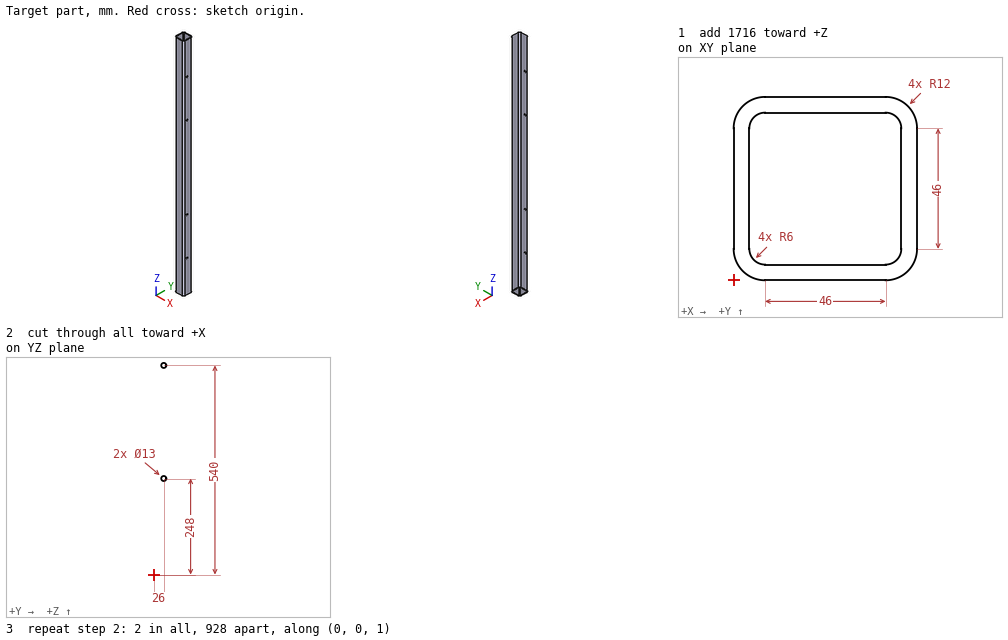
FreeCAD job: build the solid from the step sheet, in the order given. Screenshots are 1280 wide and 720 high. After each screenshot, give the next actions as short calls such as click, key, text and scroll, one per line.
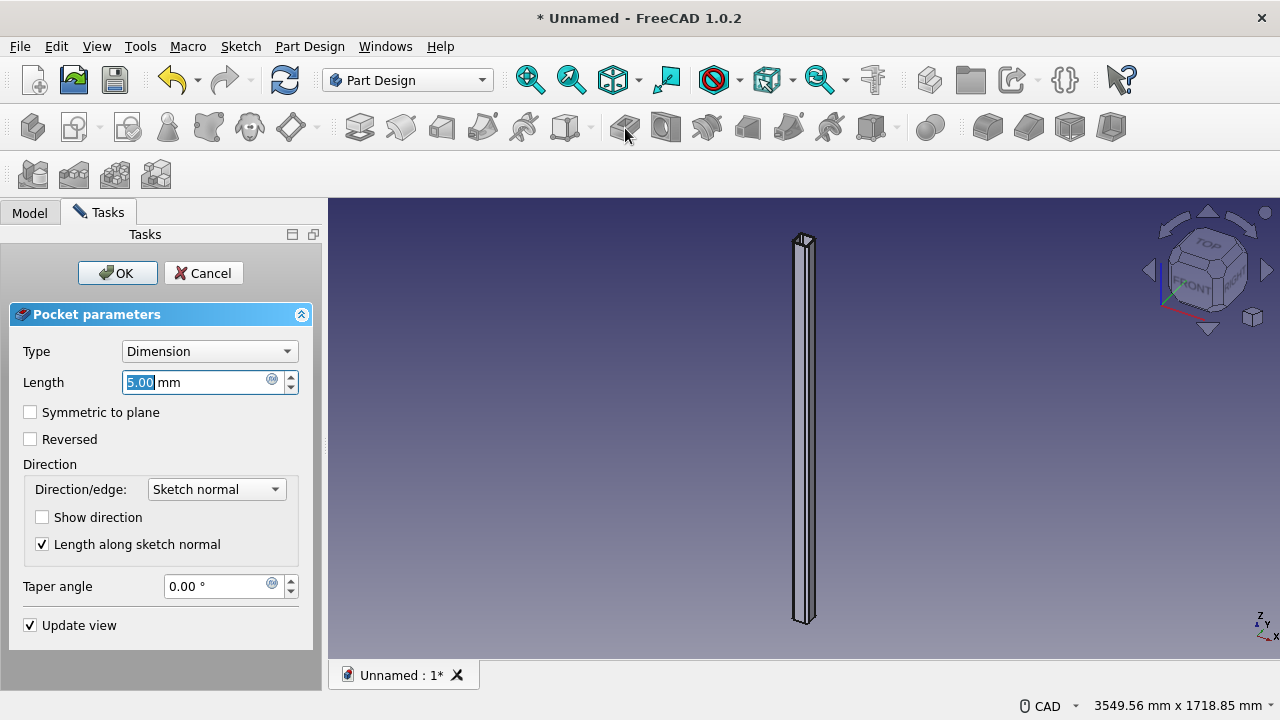
click(210, 352)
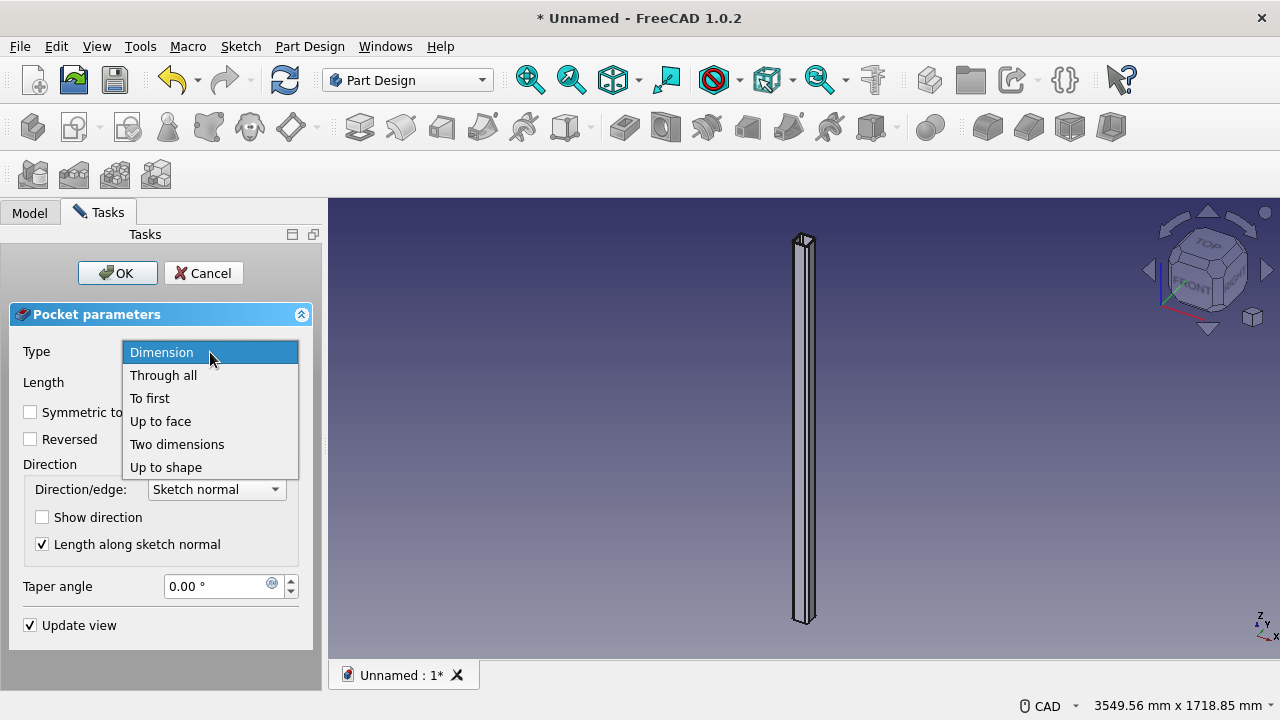
click(208, 376)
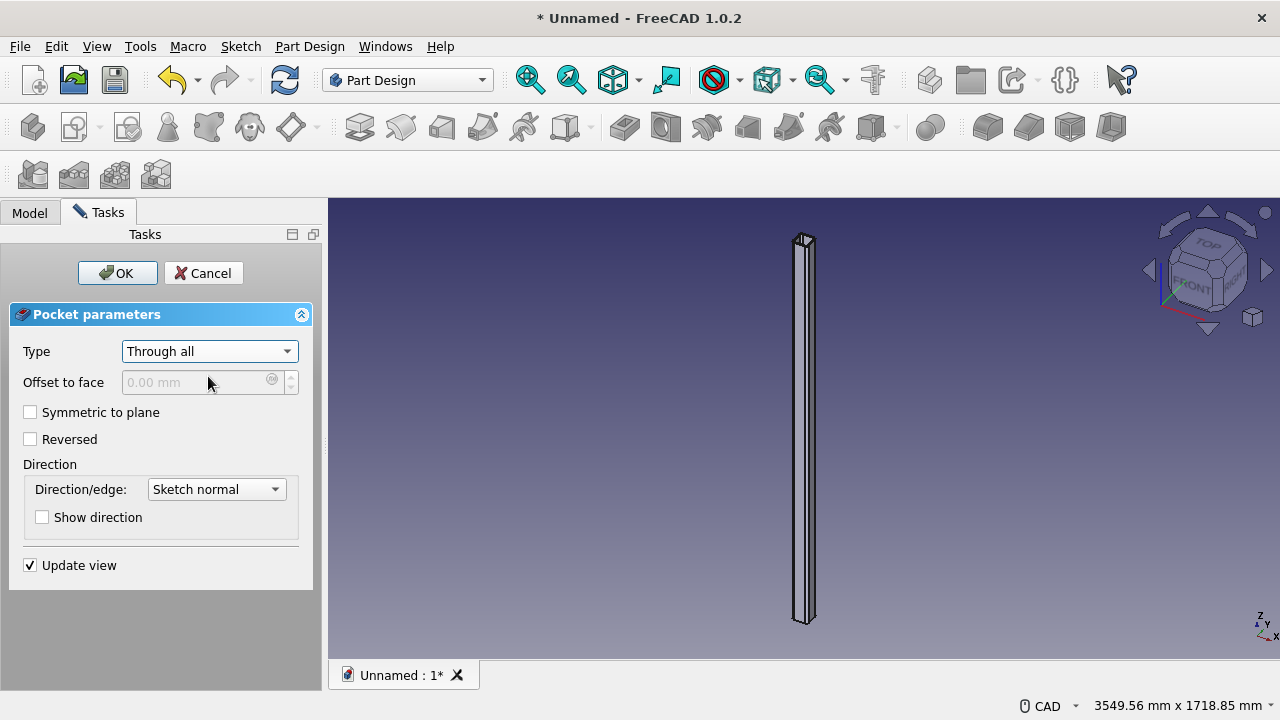
click(31, 439)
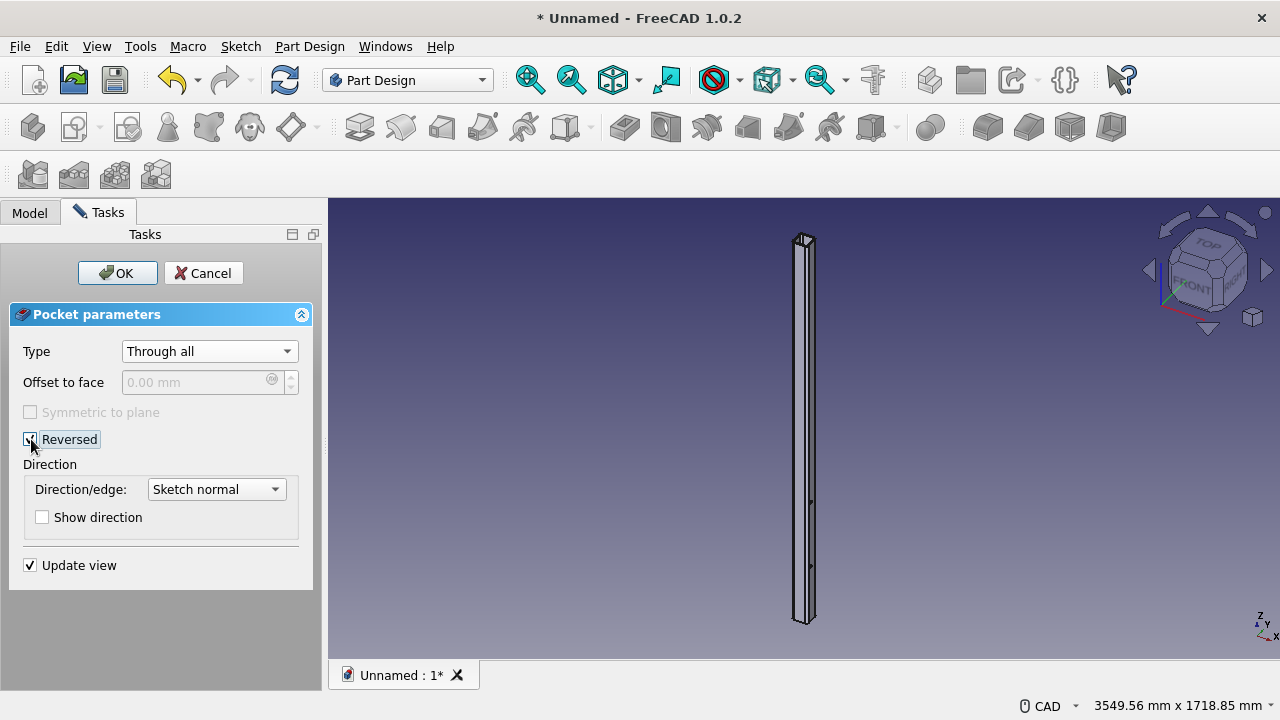
click(118, 273)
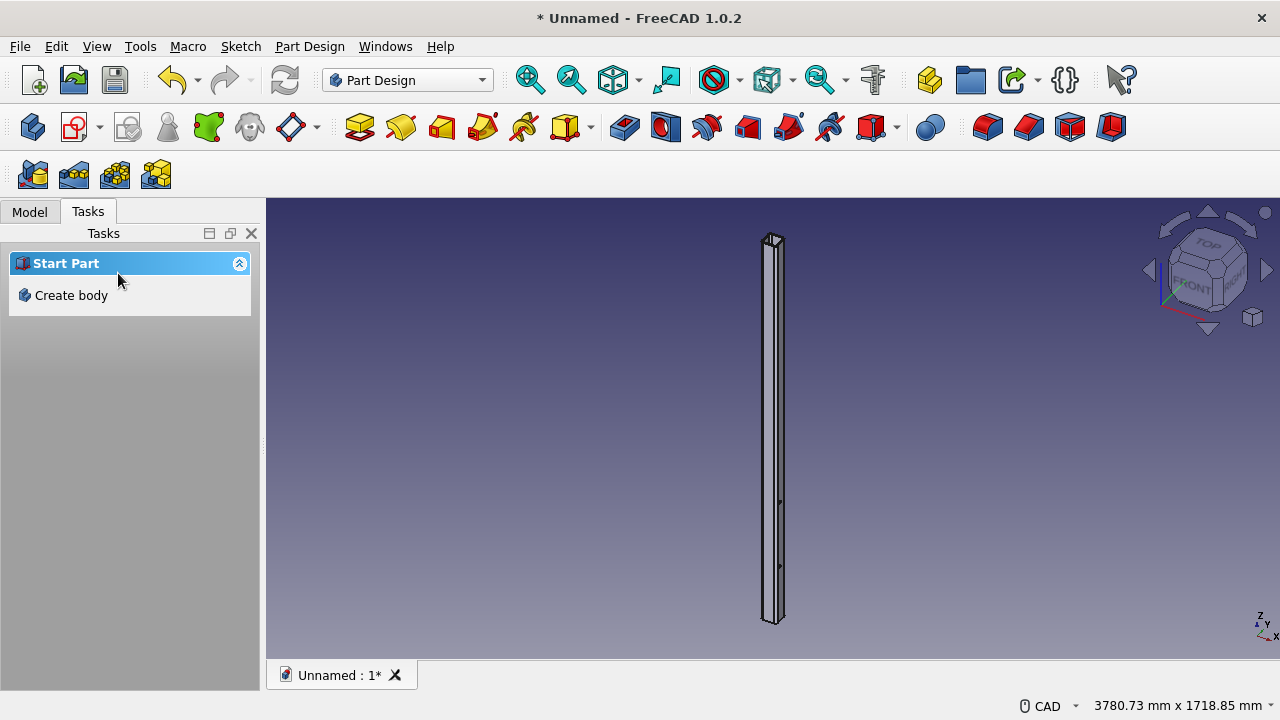
click(30, 212)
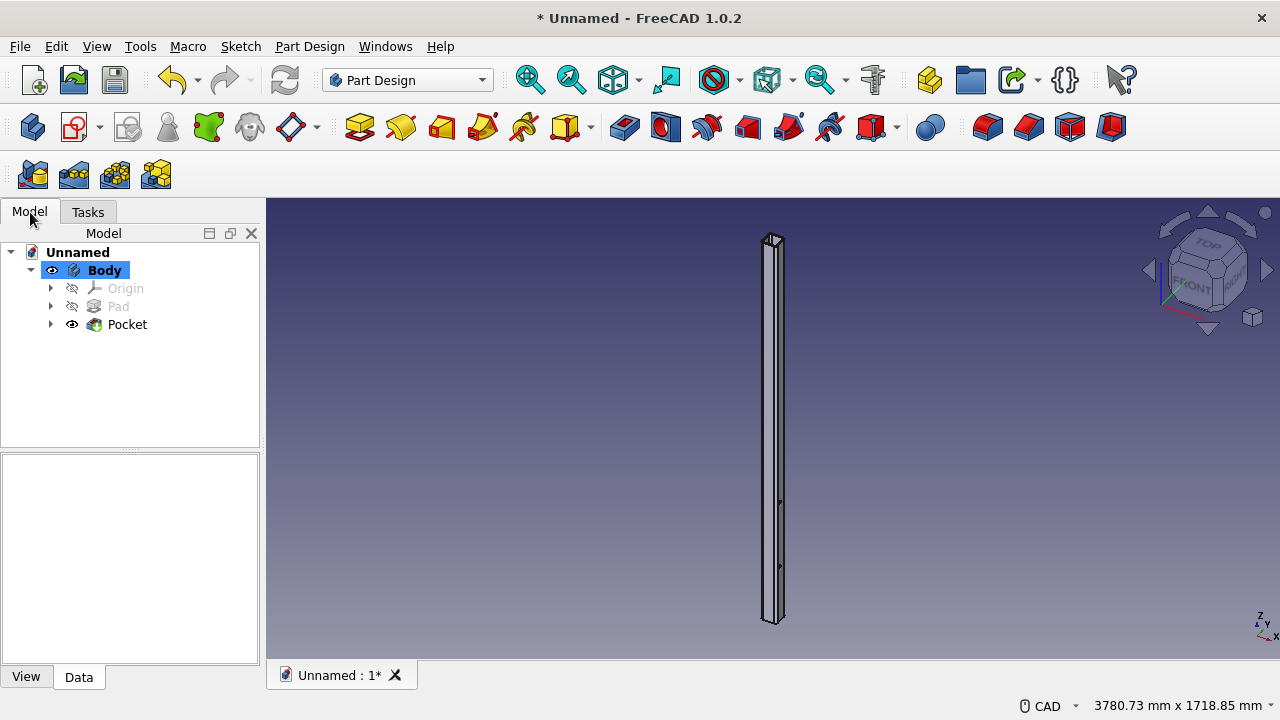
click(117, 324)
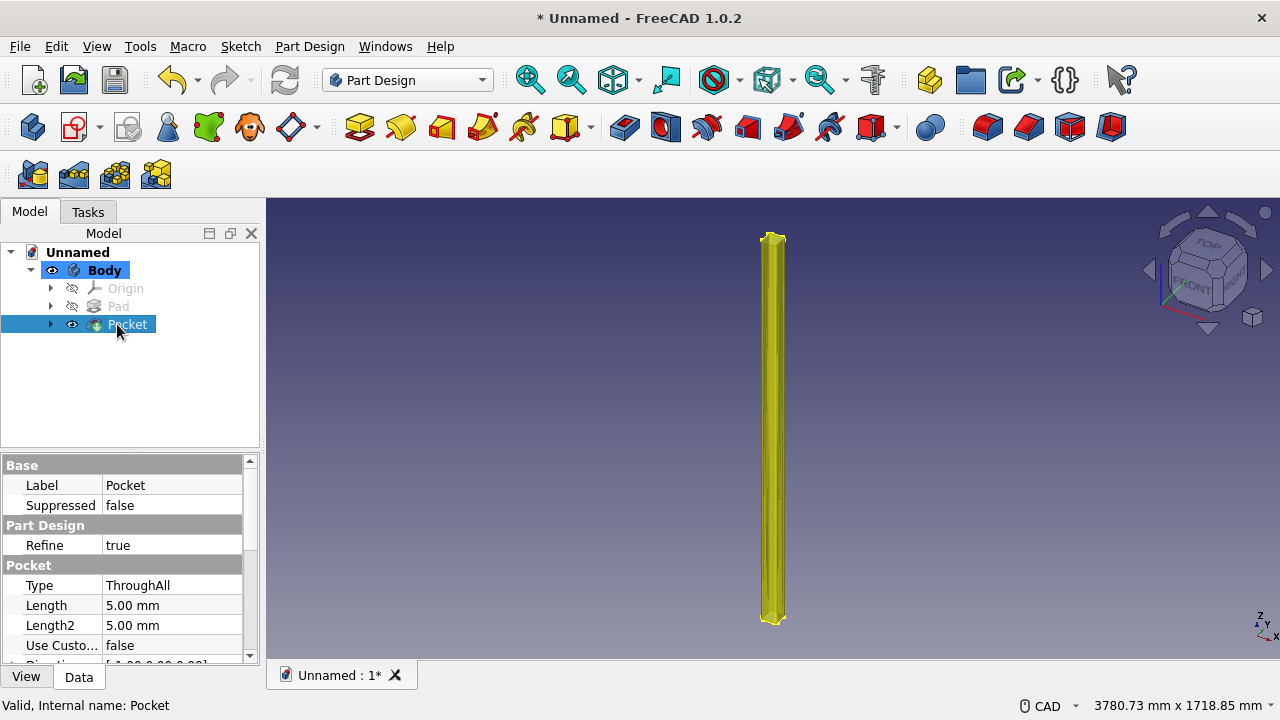
click(74, 174)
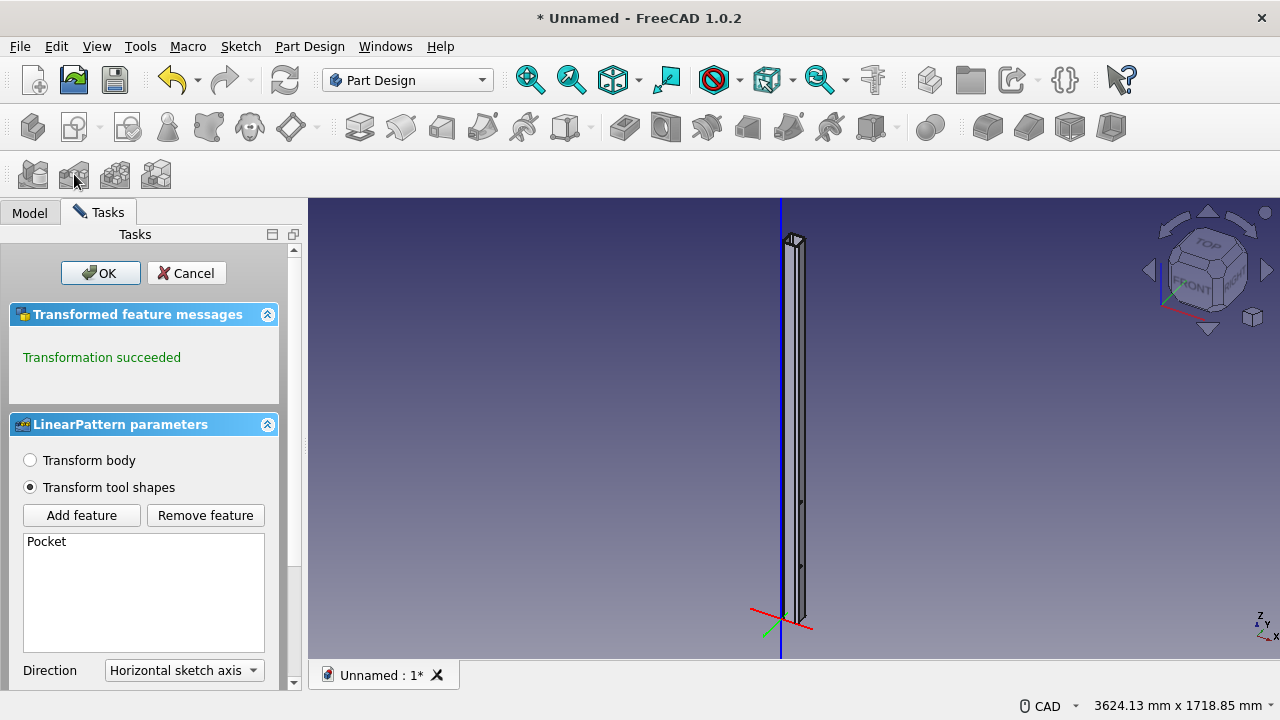
click(185, 670)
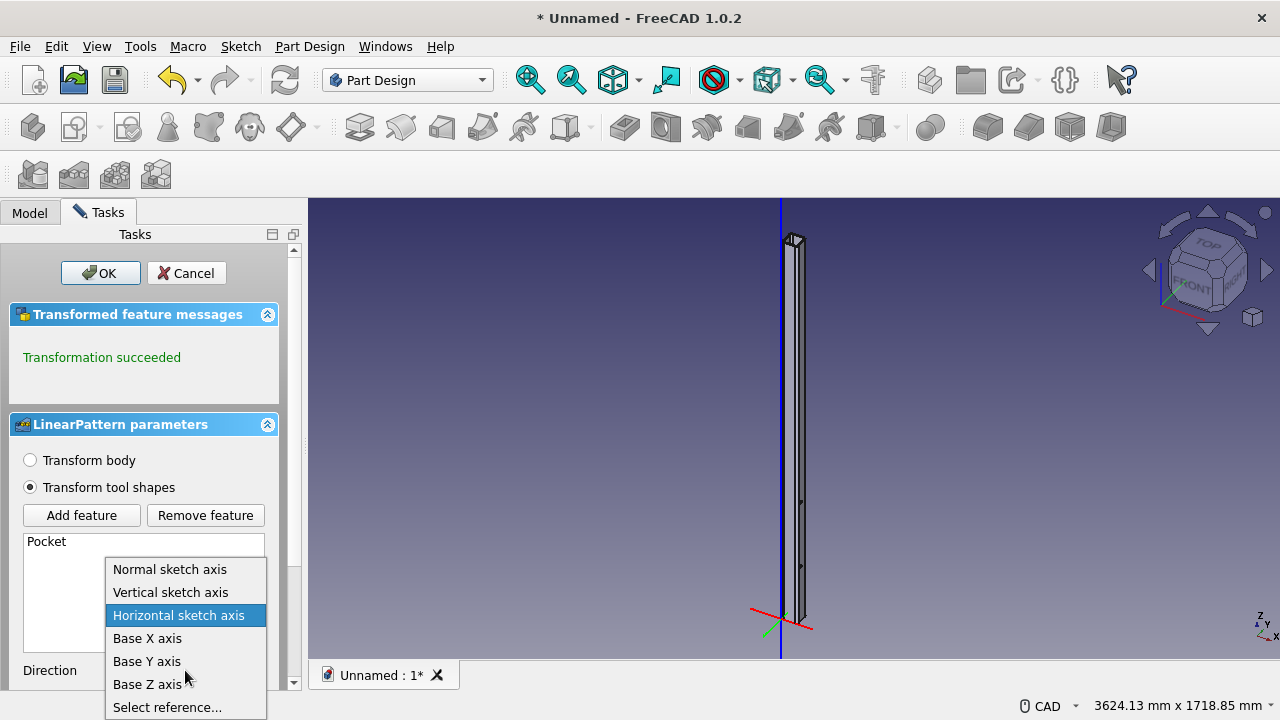
click(184, 684)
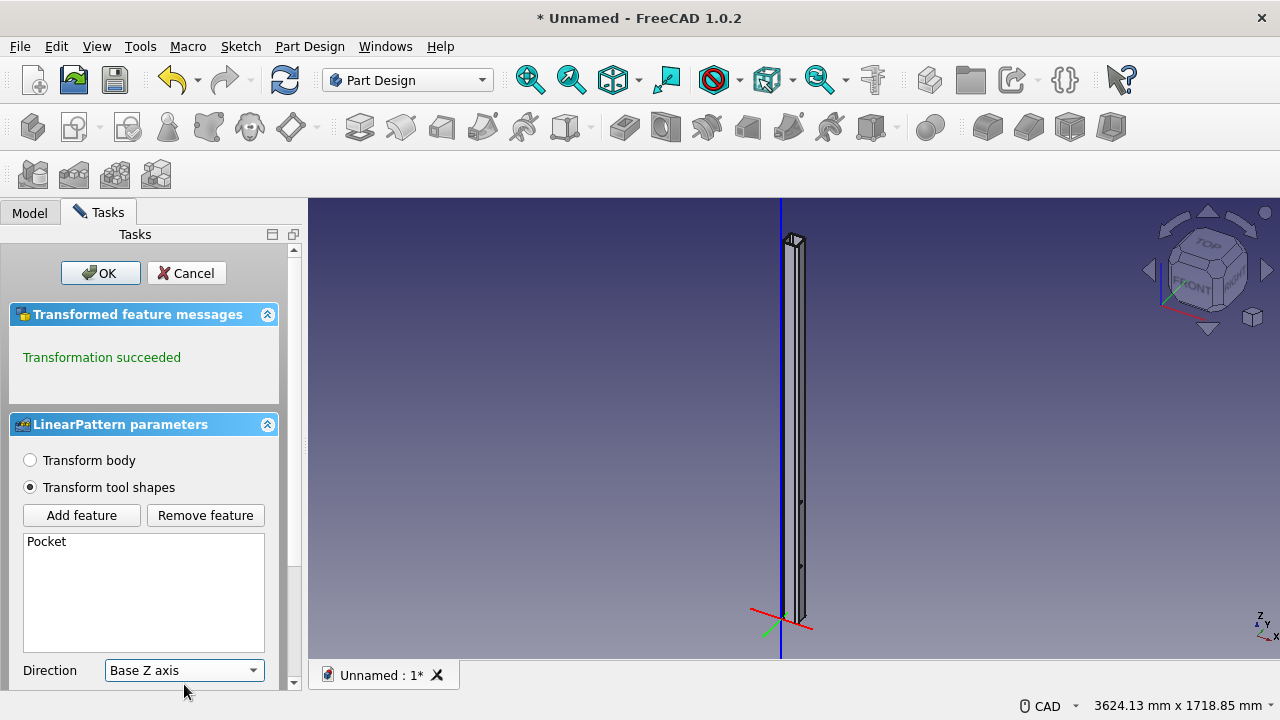
scroll(294, 467, down, 2)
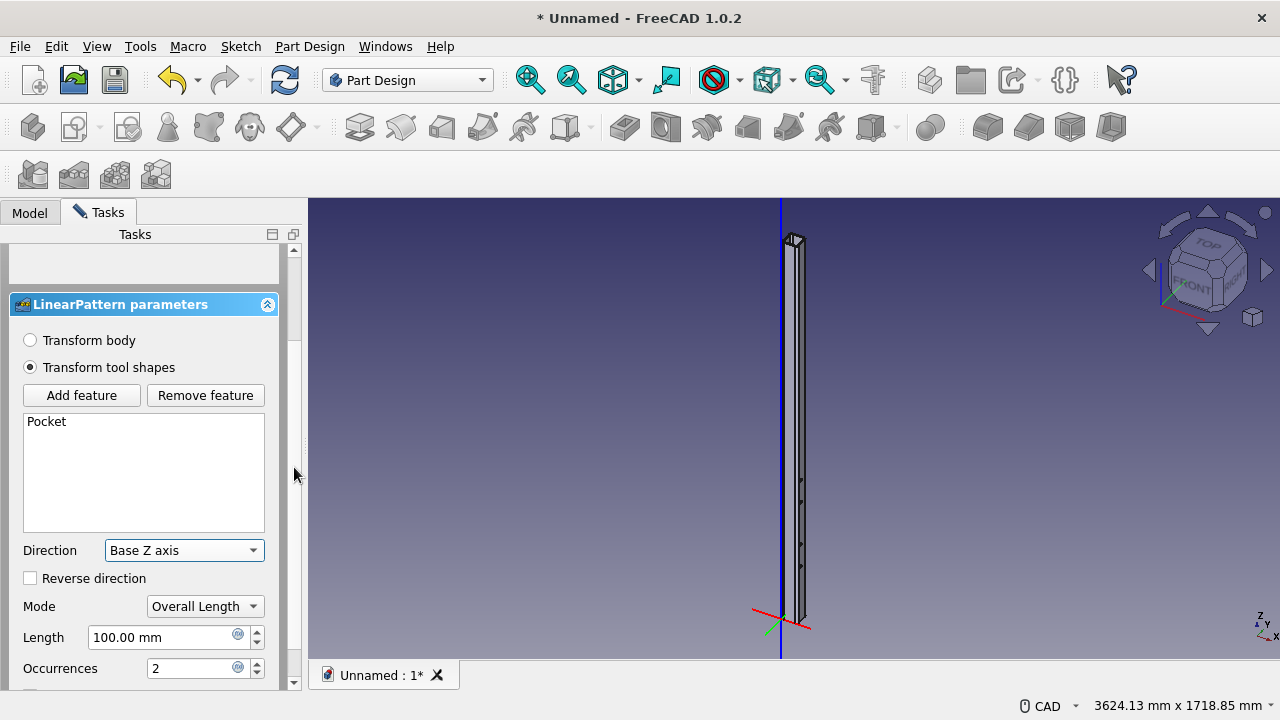
click(206, 606)